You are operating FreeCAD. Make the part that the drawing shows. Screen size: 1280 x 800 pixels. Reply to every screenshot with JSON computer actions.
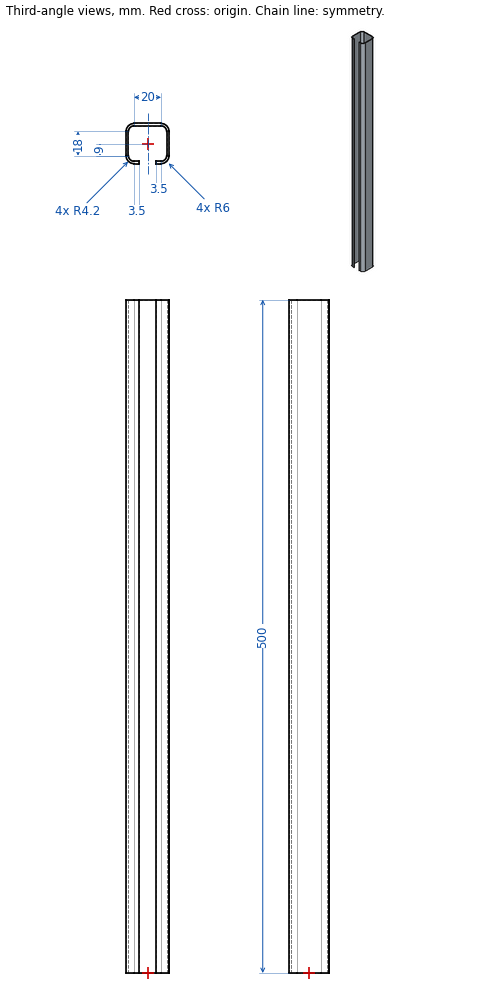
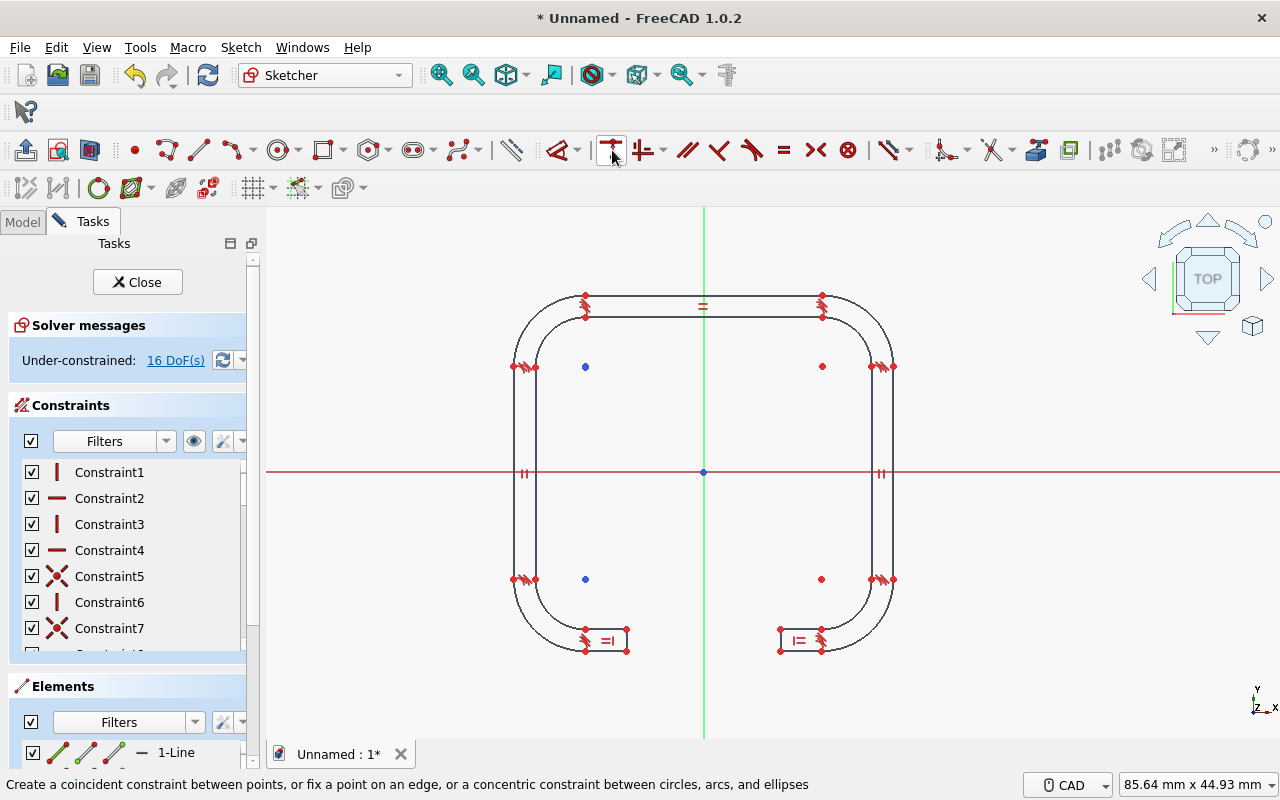
{"action": "left_click", "coordinate": [563, 323]}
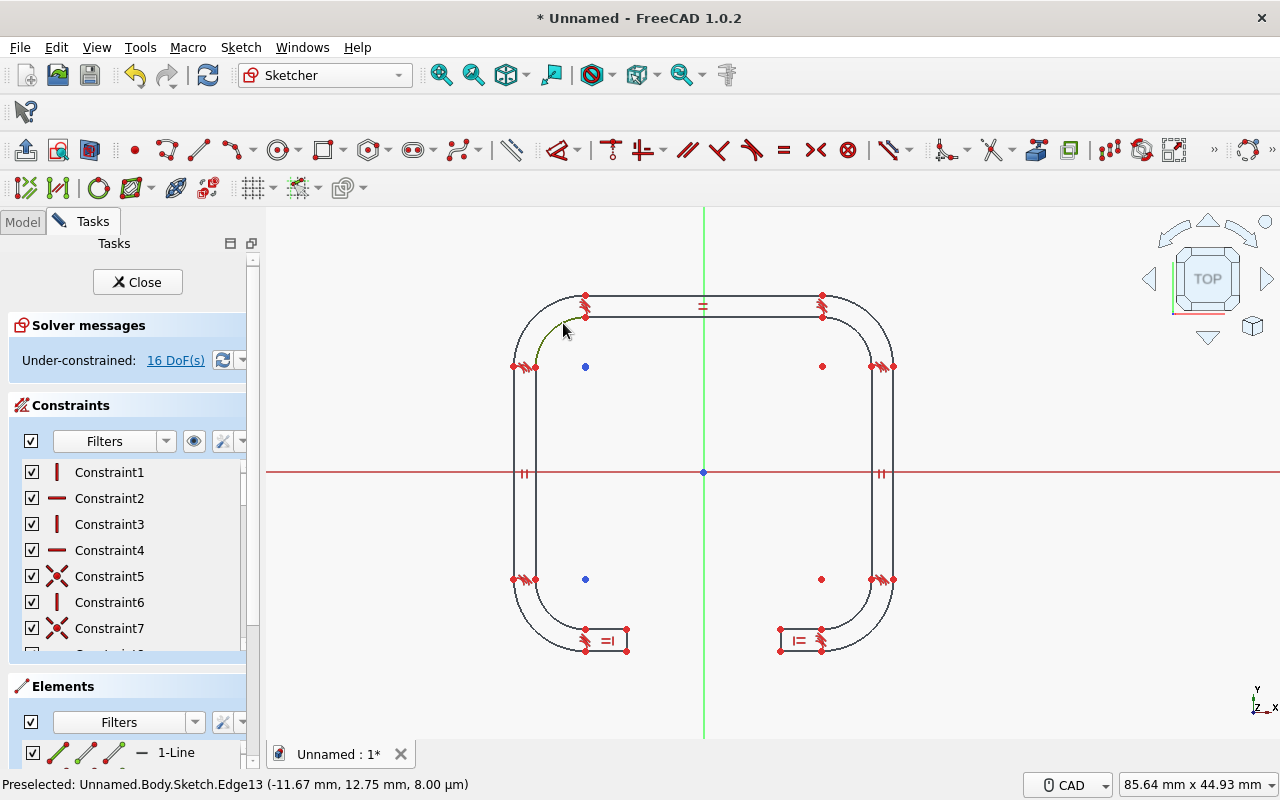
{"action": "left_click", "coordinate": [553, 303]}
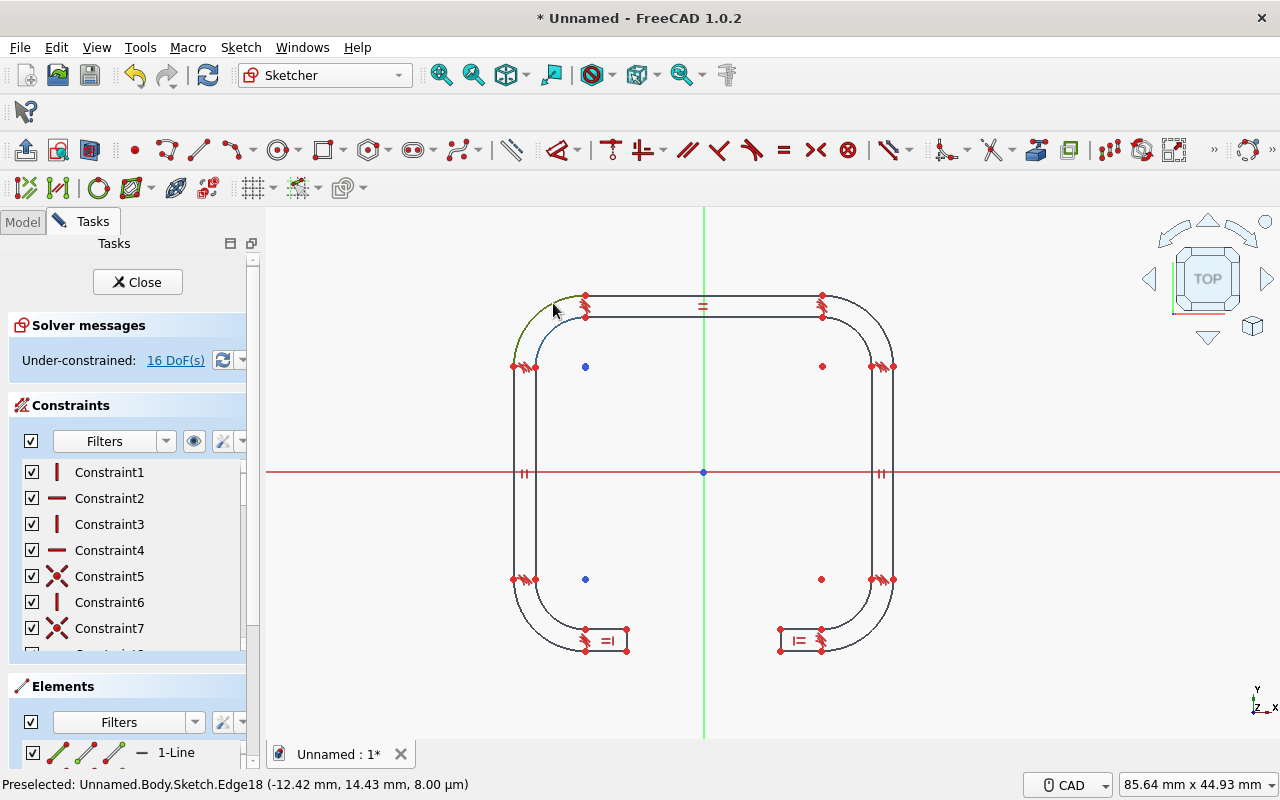
{"action": "left_click", "coordinate": [612, 150]}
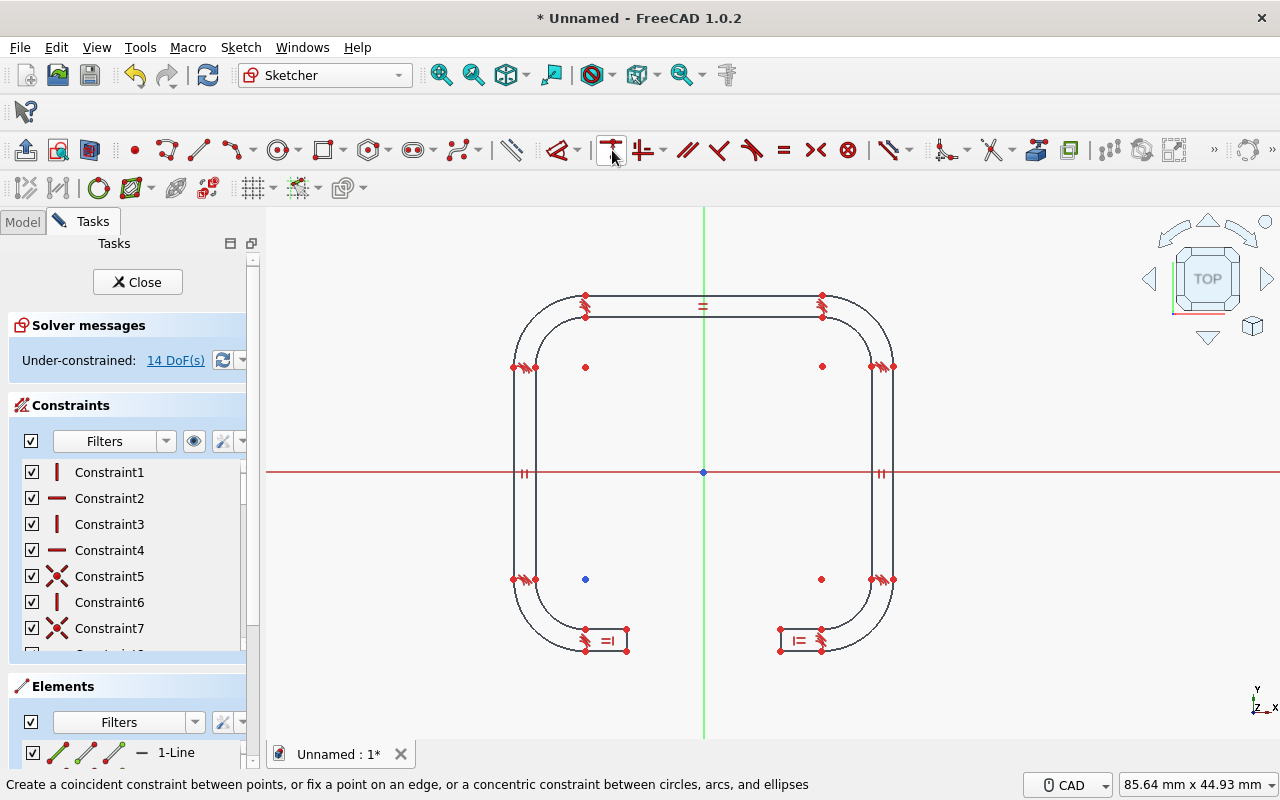
{"action": "left_click", "coordinate": [522, 612]}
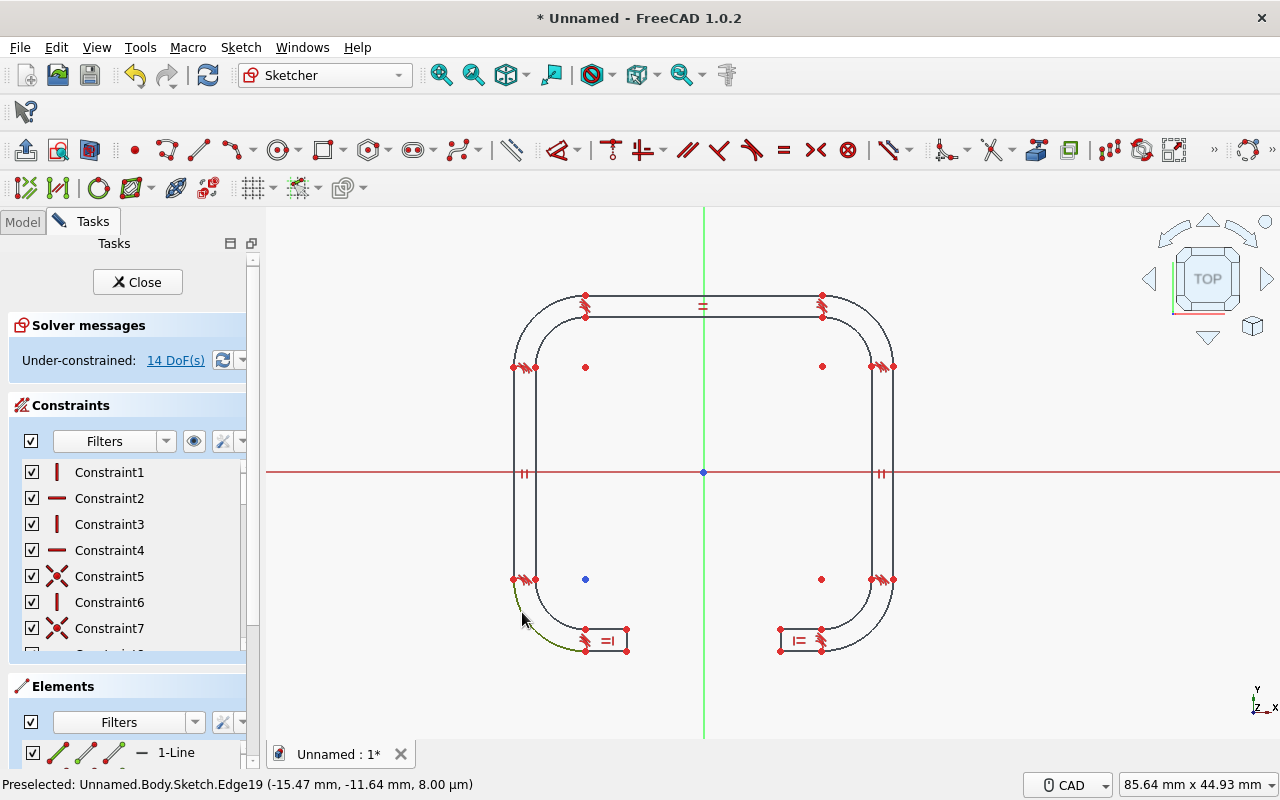
{"action": "left_click", "coordinate": [541, 602]}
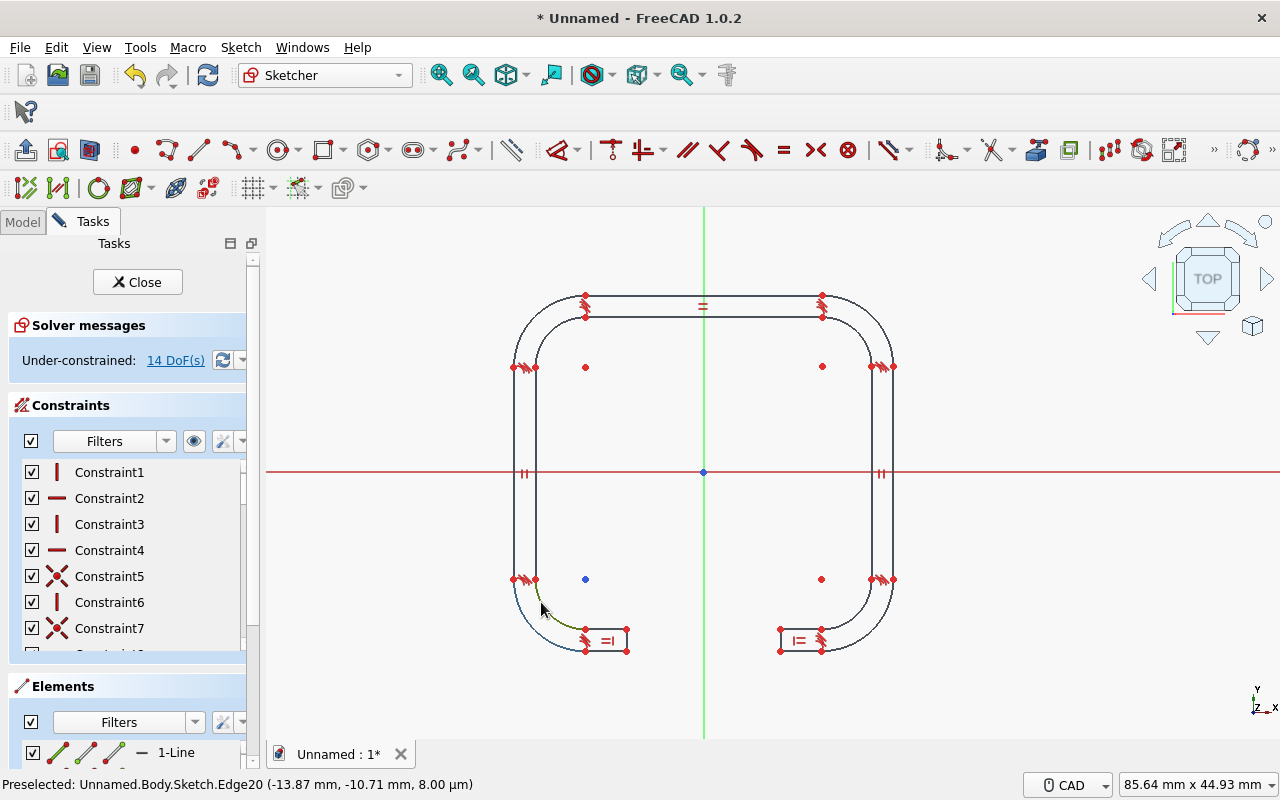
{"action": "left_click", "coordinate": [612, 150]}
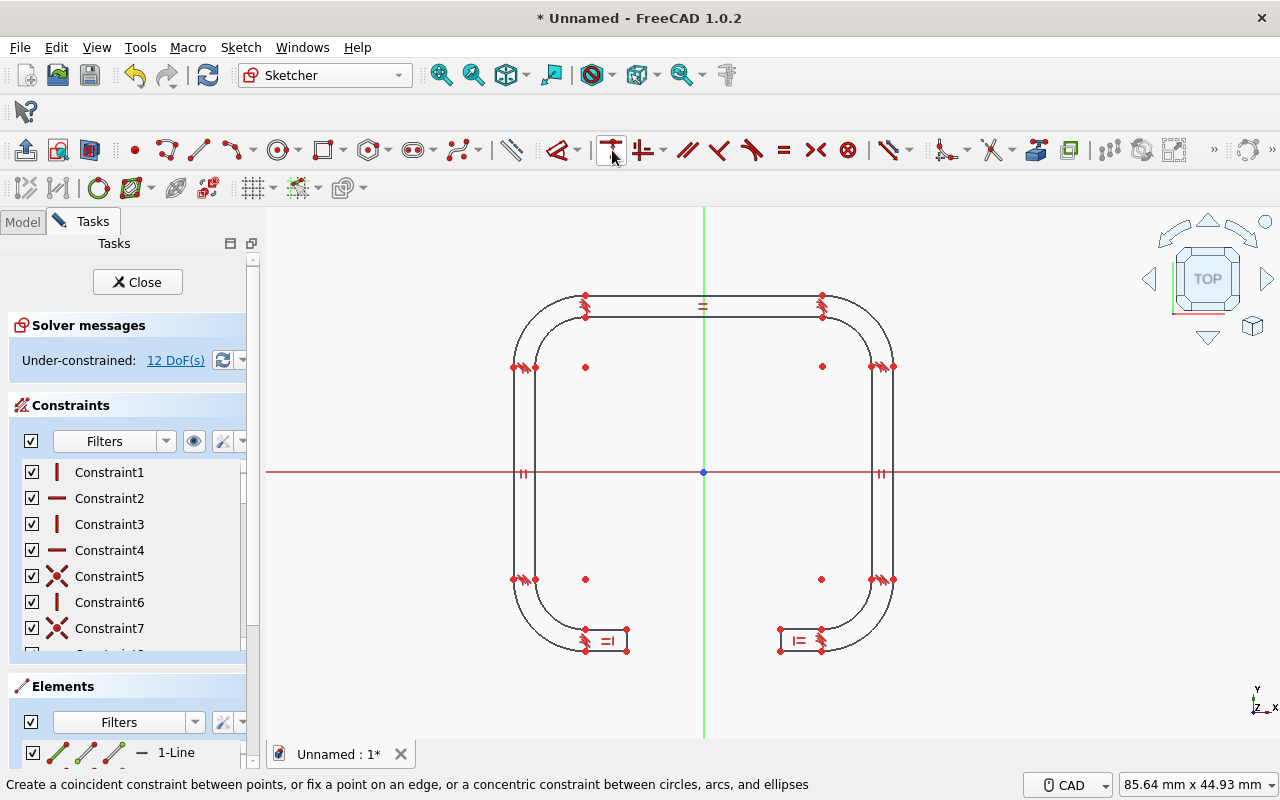
{"action": "left_click", "coordinate": [563, 323]}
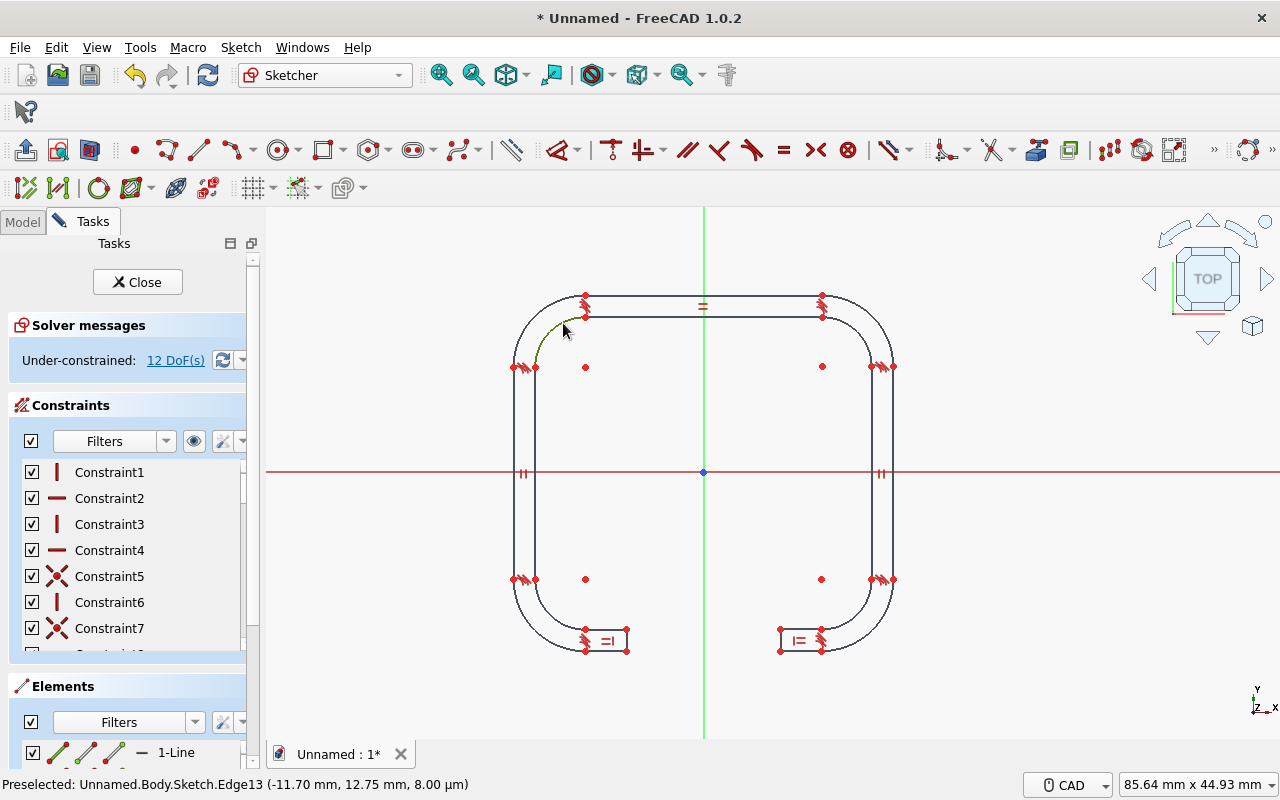
{"action": "left_click", "coordinate": [866, 344]}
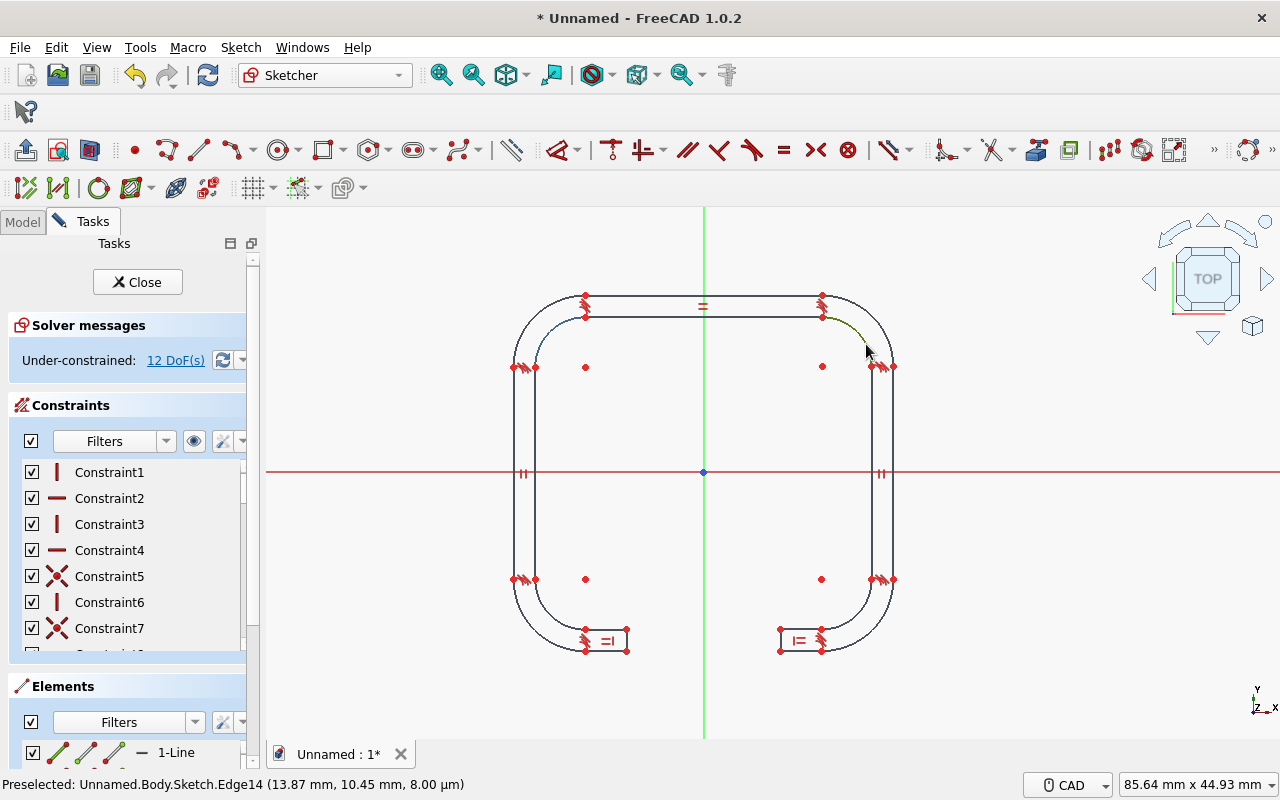
{"action": "left_click", "coordinate": [844, 624]}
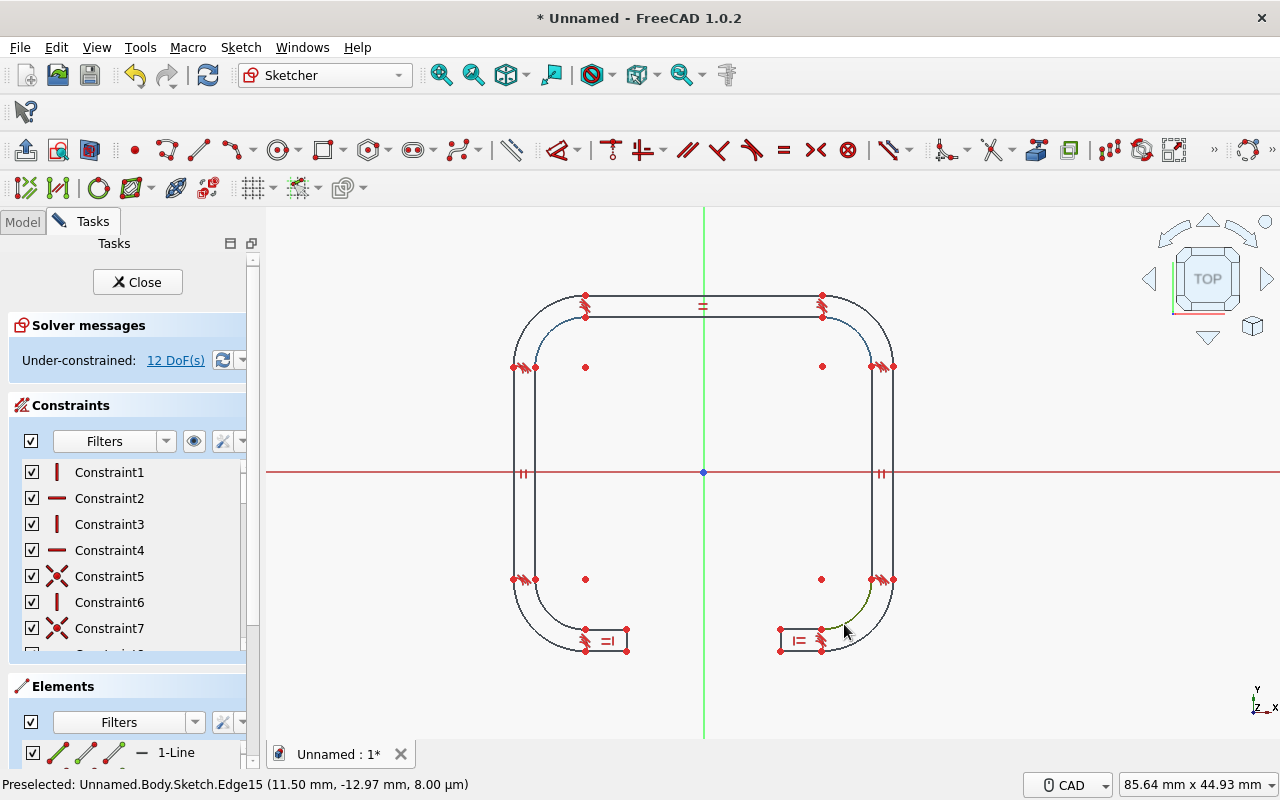
{"action": "left_click", "coordinate": [541, 602]}